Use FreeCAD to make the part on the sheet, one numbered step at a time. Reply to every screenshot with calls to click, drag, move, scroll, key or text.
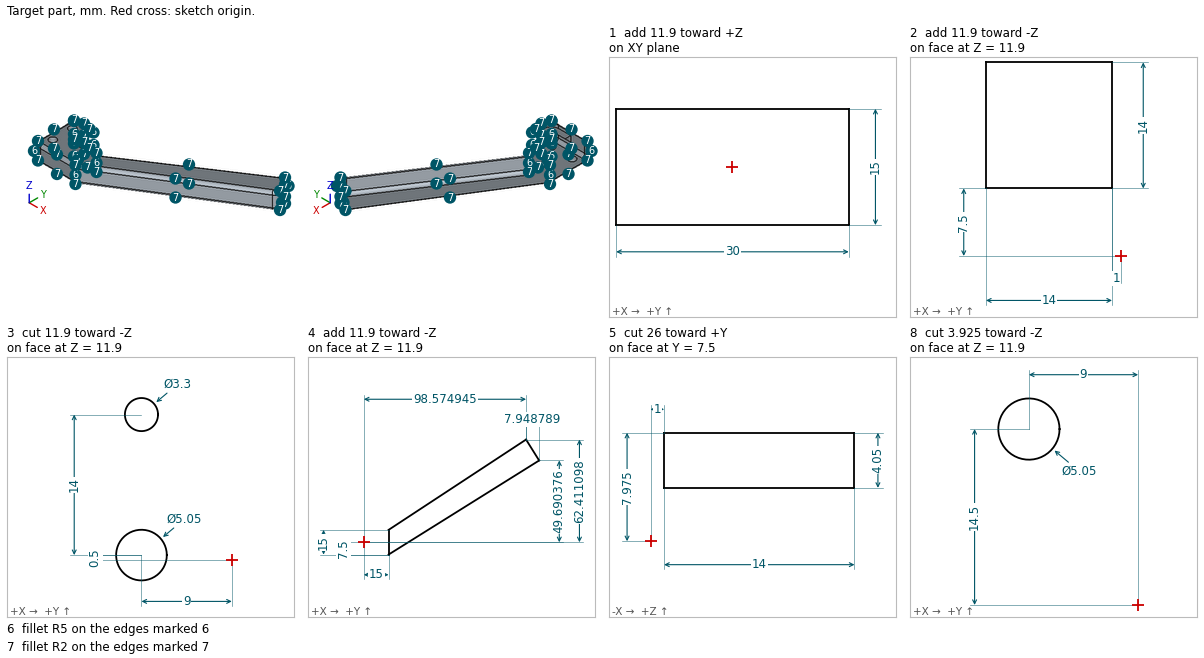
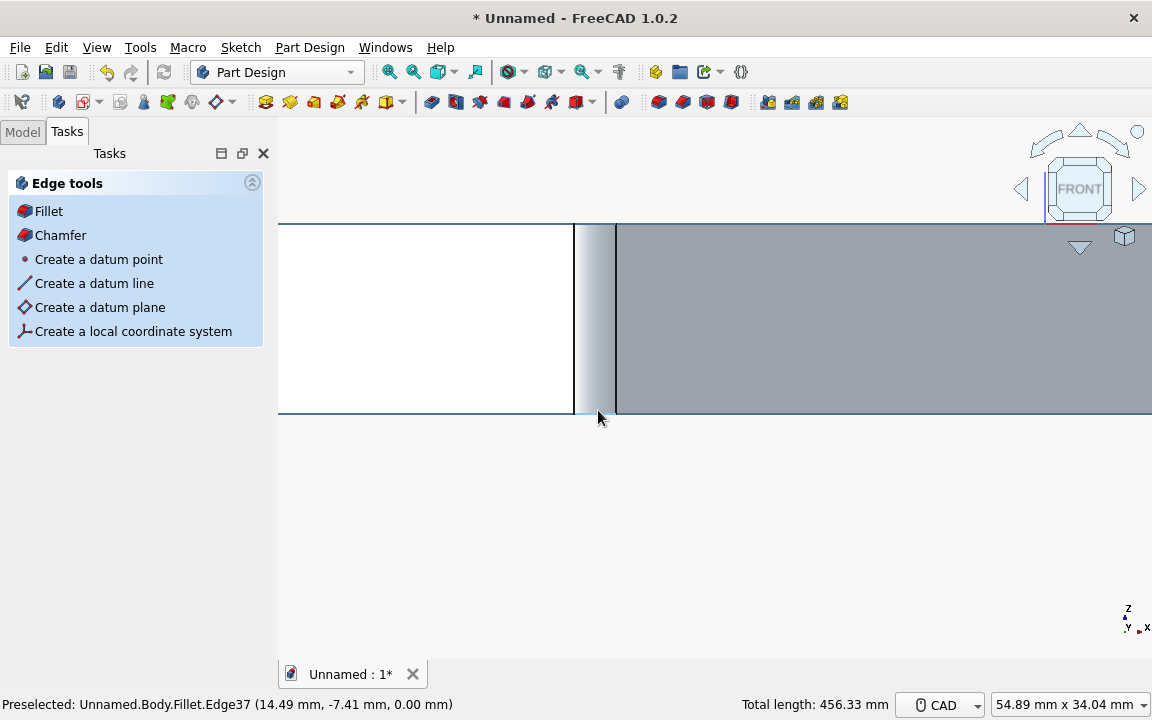
key(v)
key(f)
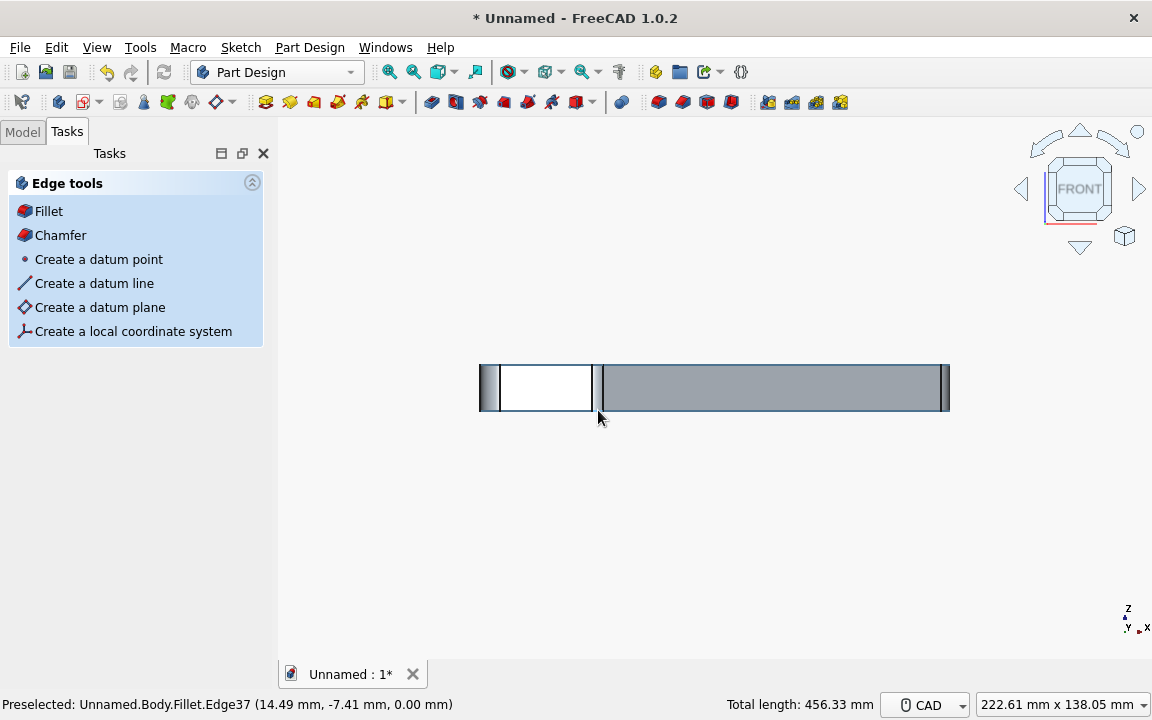
key(3)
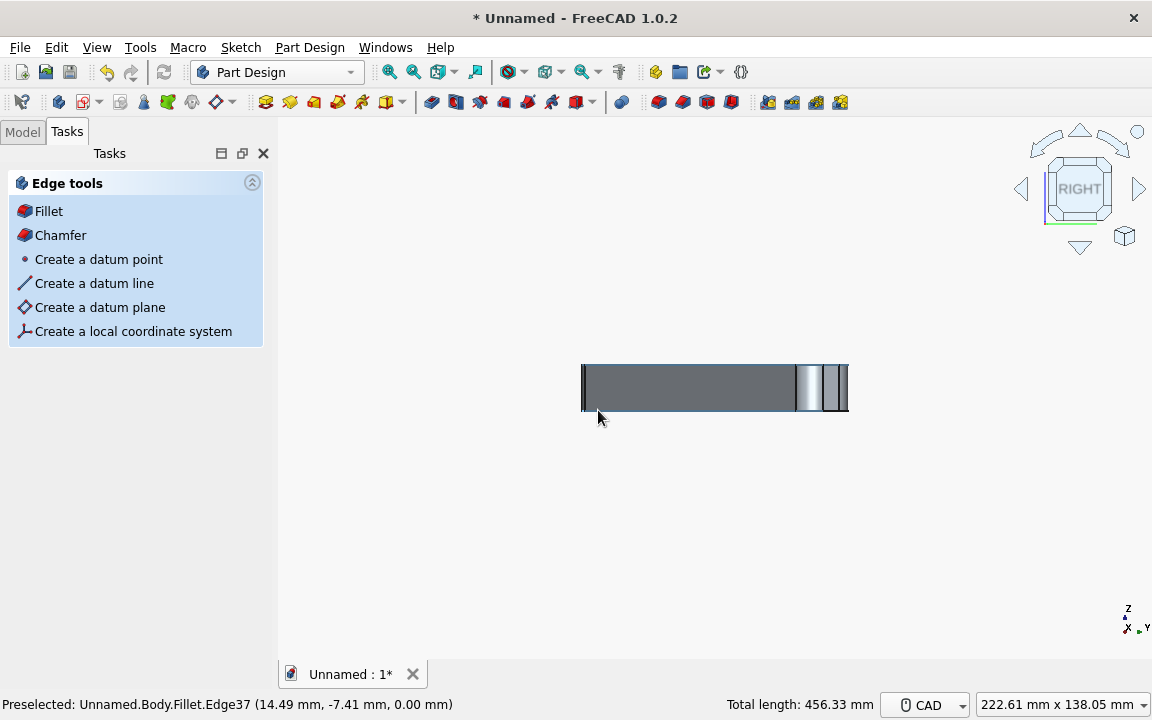
click(390, 72)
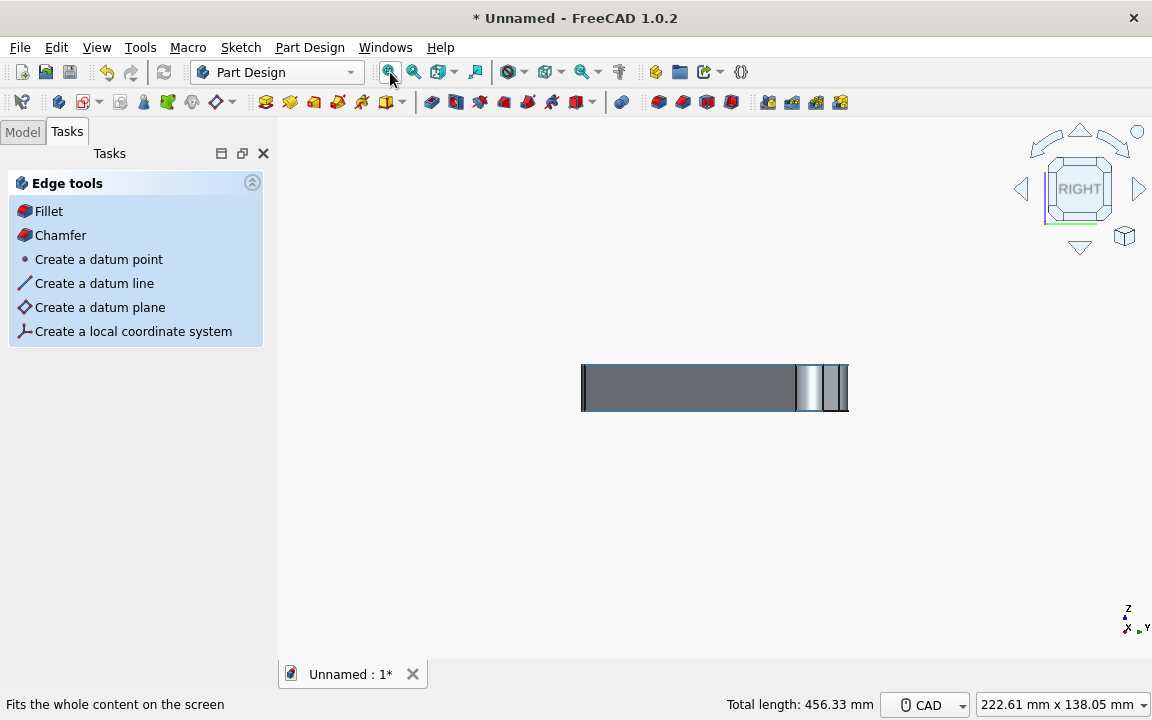
click(831, 410, ctrl)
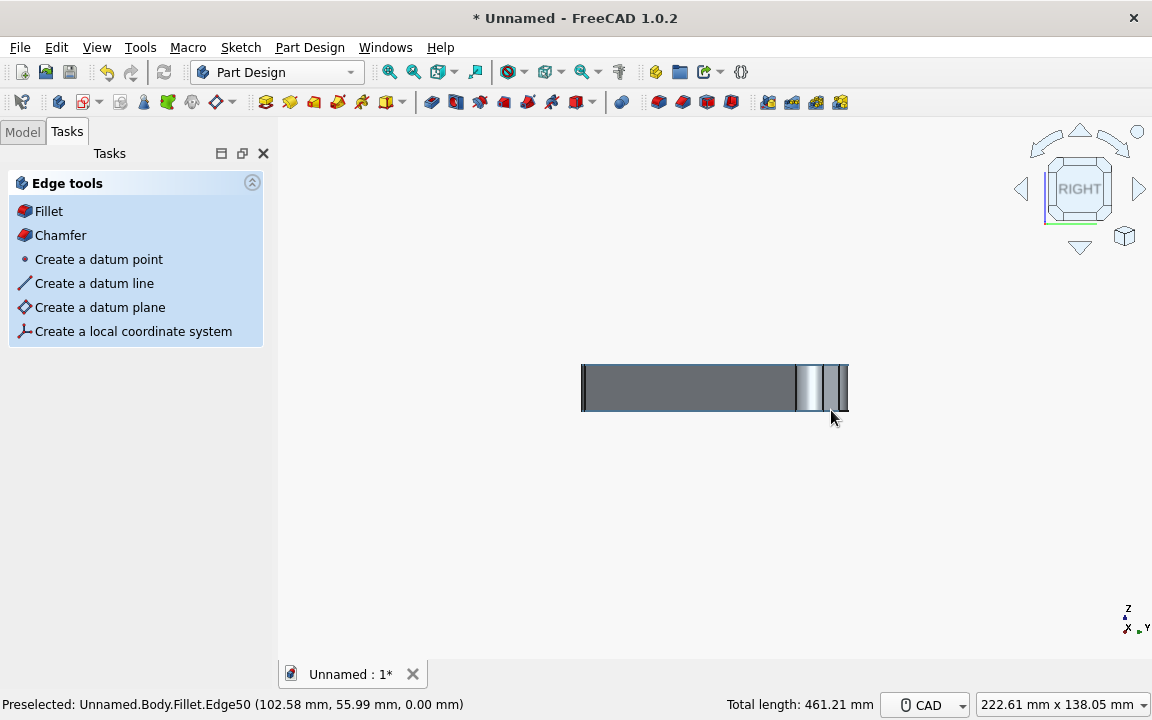
click(848, 410, ctrl)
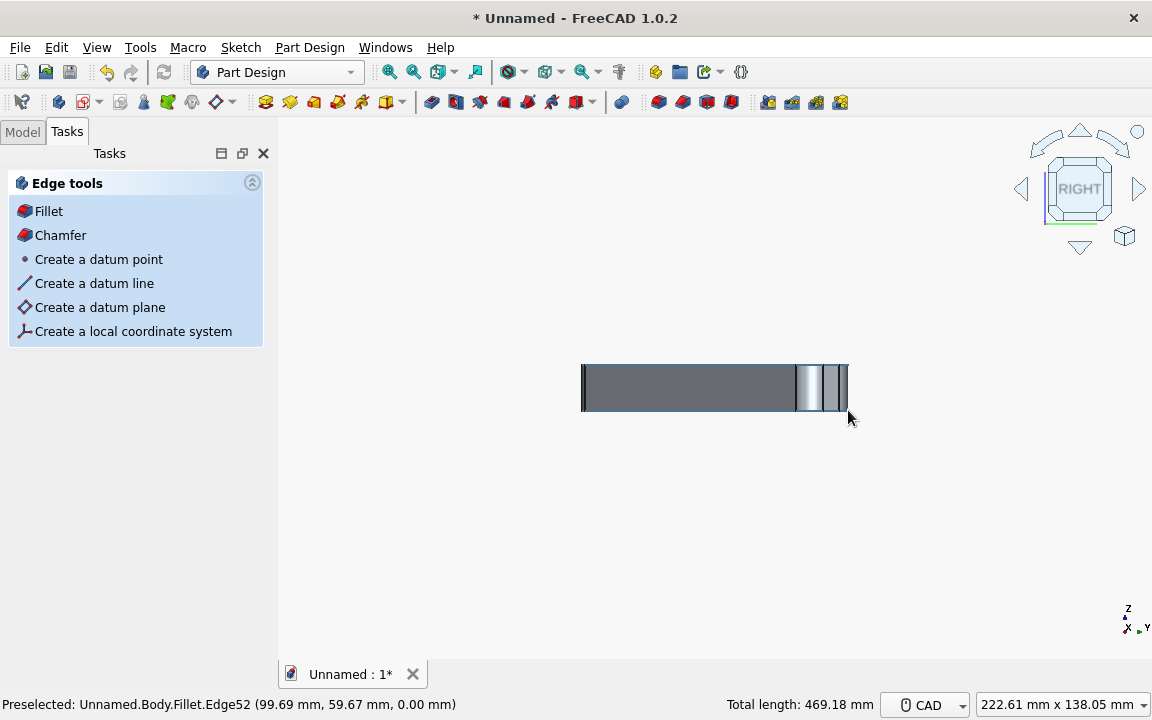
scroll(641, 410, up, 7)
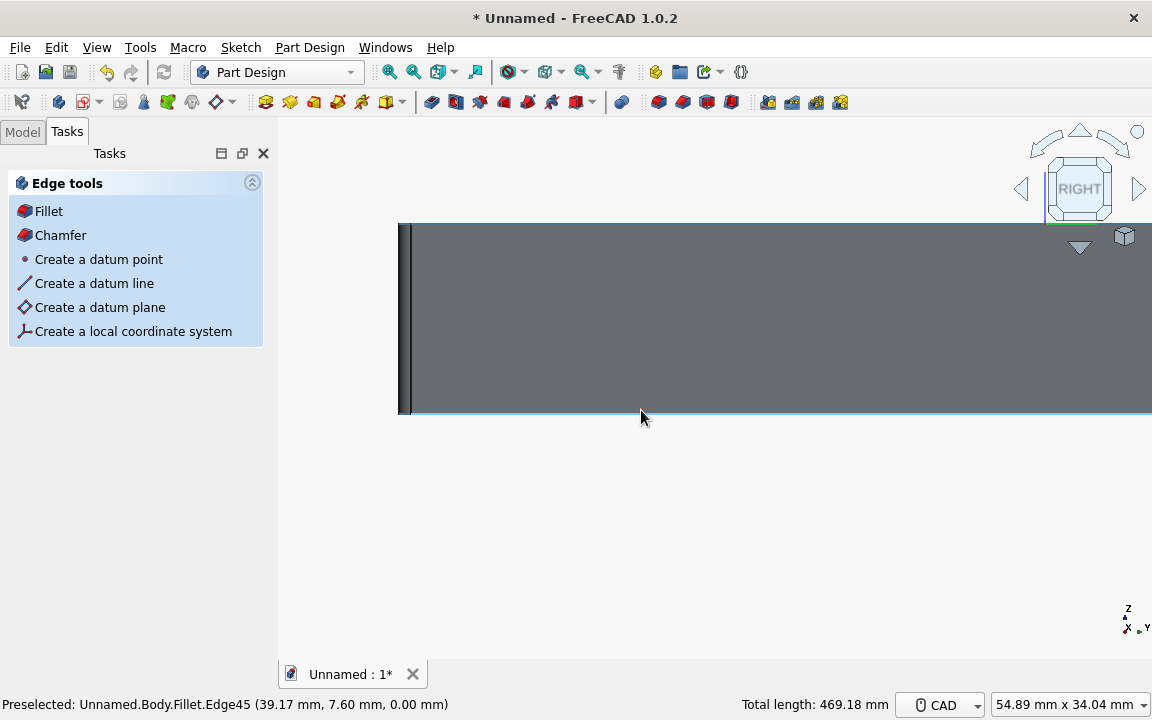
click(390, 72)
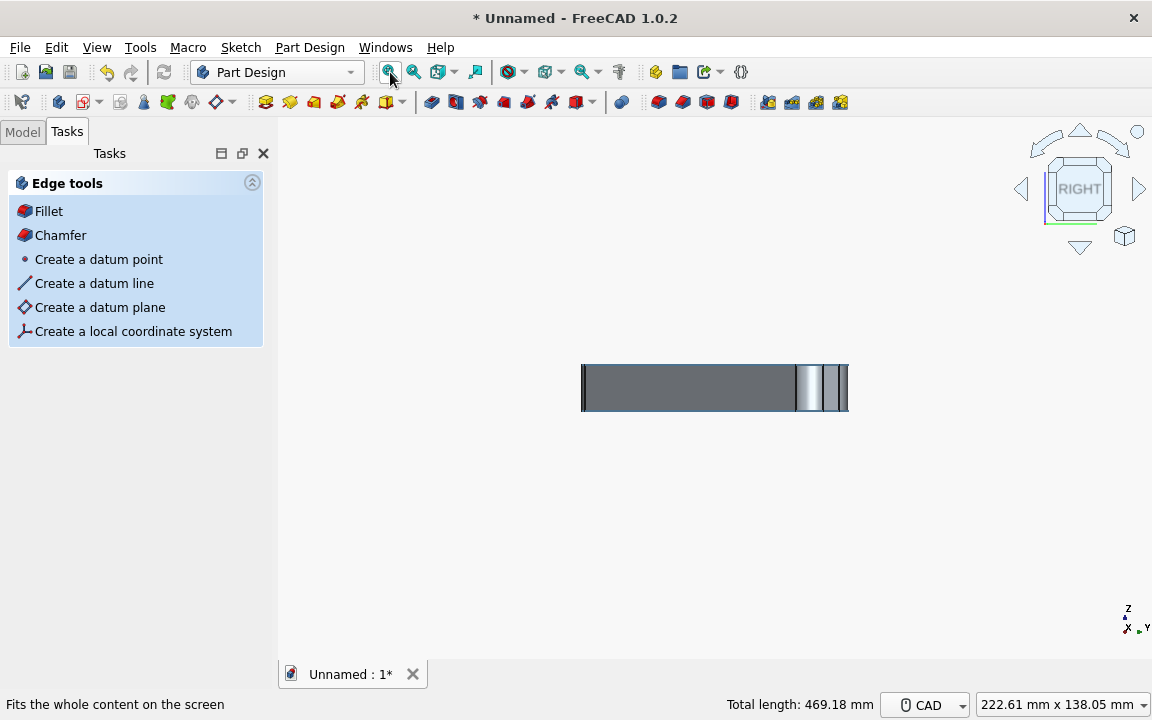
key(5)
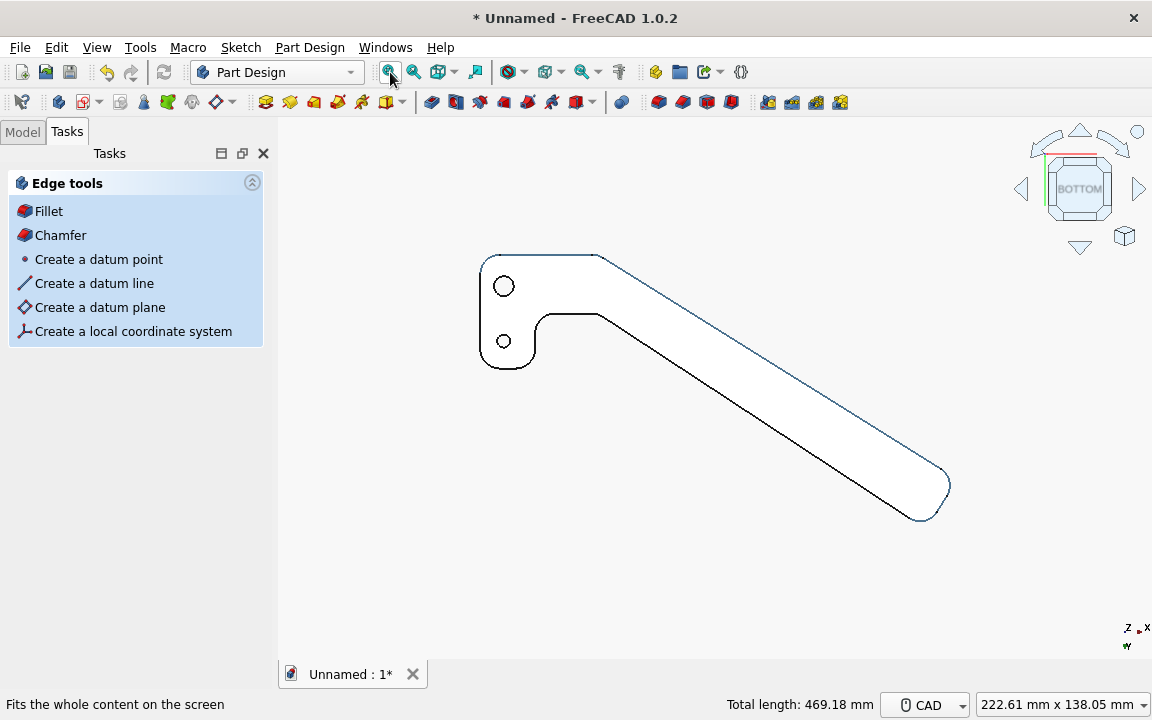
click(594, 313, ctrl)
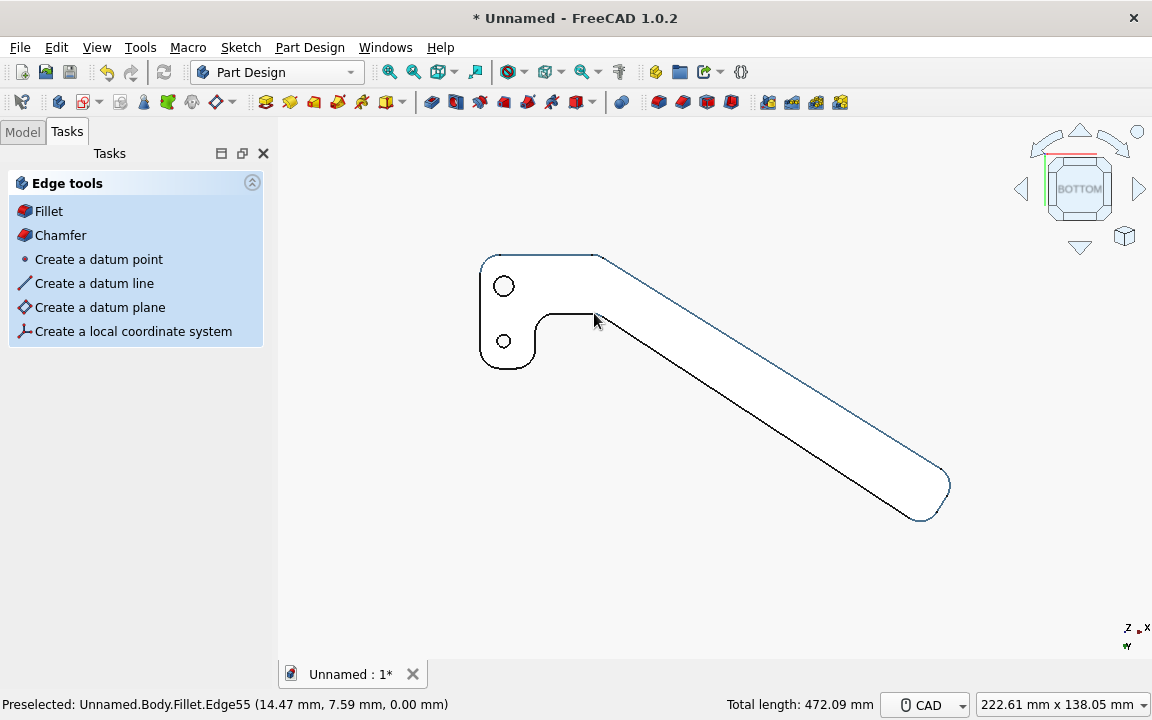
click(539, 321, ctrl)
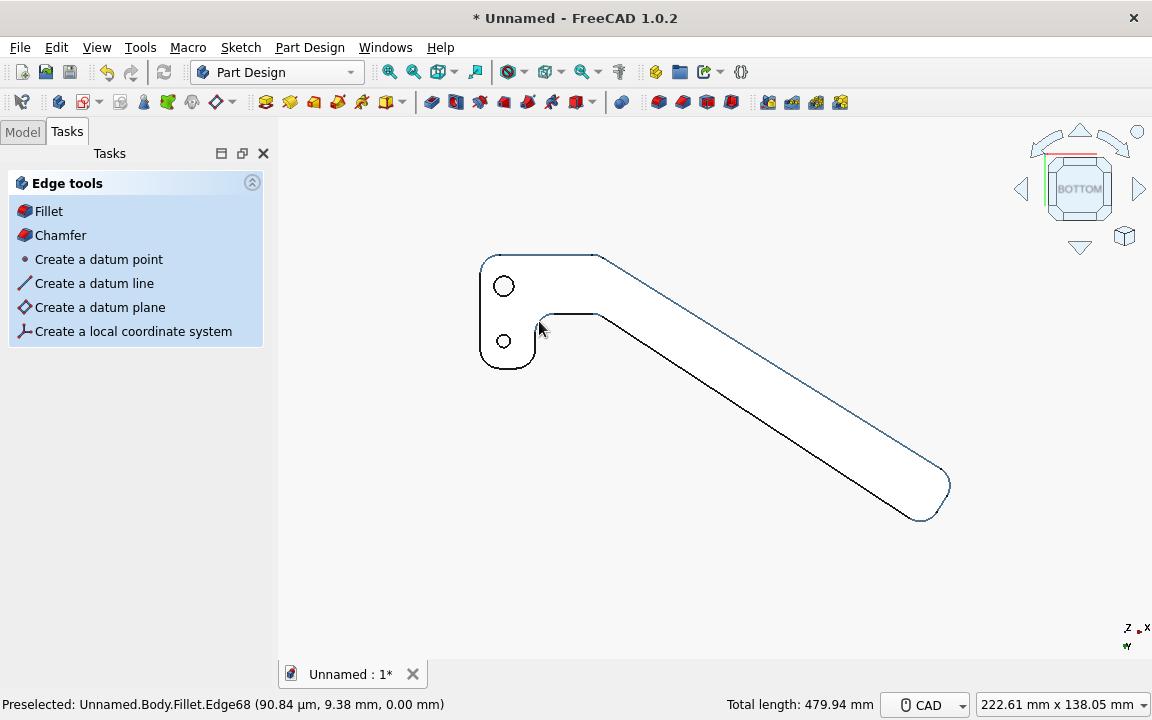
click(756, 416, ctrl)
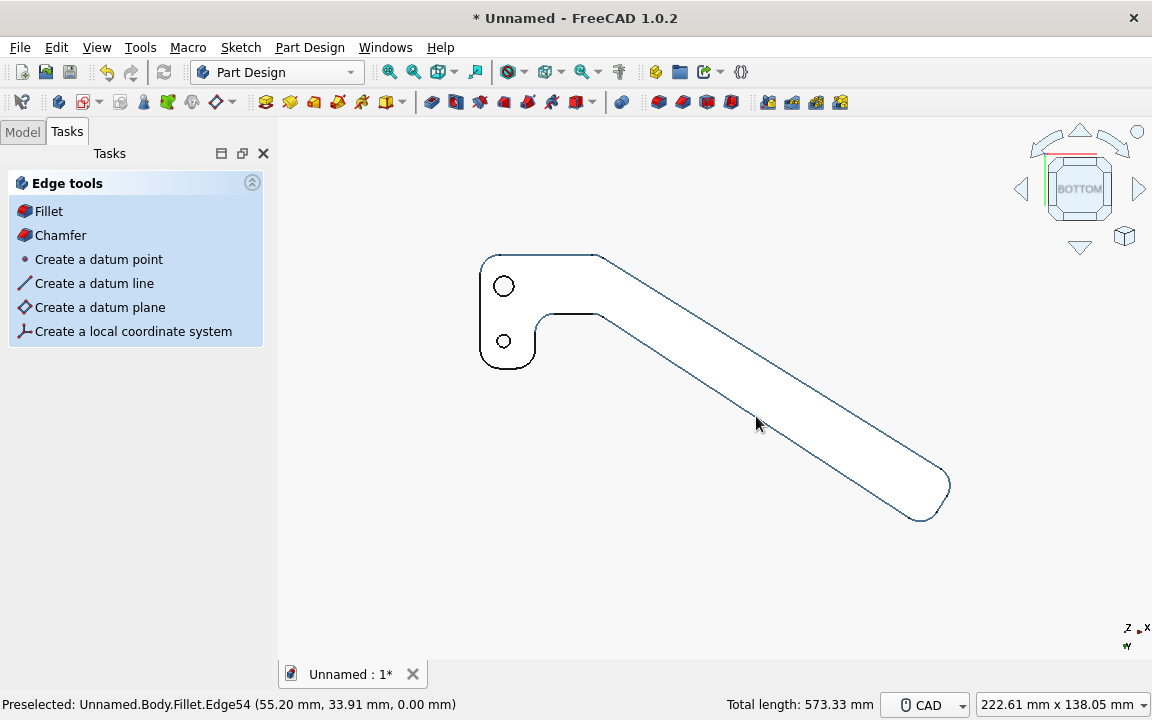
click(573, 313, ctrl)